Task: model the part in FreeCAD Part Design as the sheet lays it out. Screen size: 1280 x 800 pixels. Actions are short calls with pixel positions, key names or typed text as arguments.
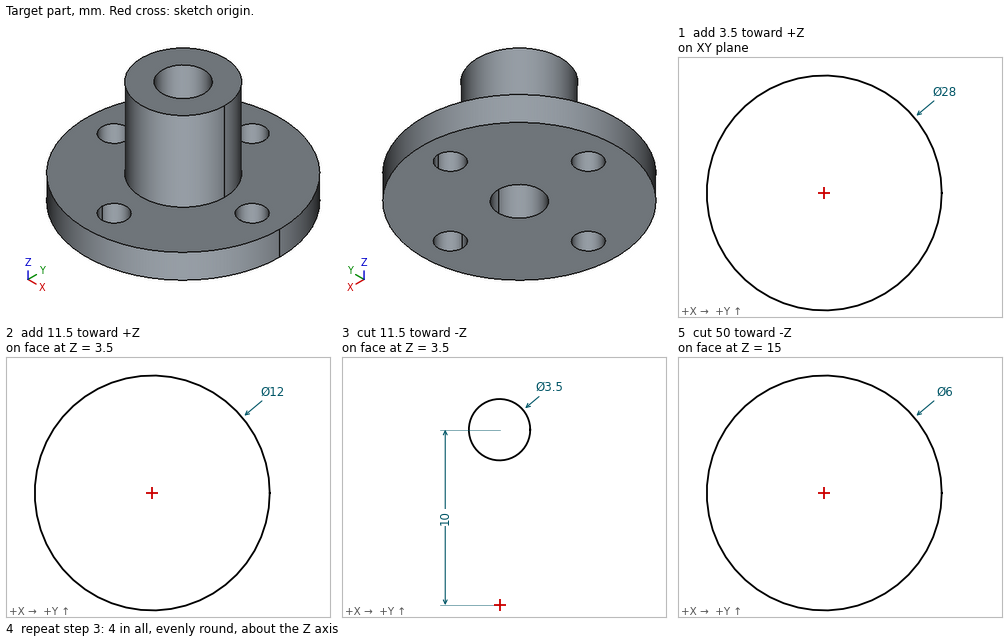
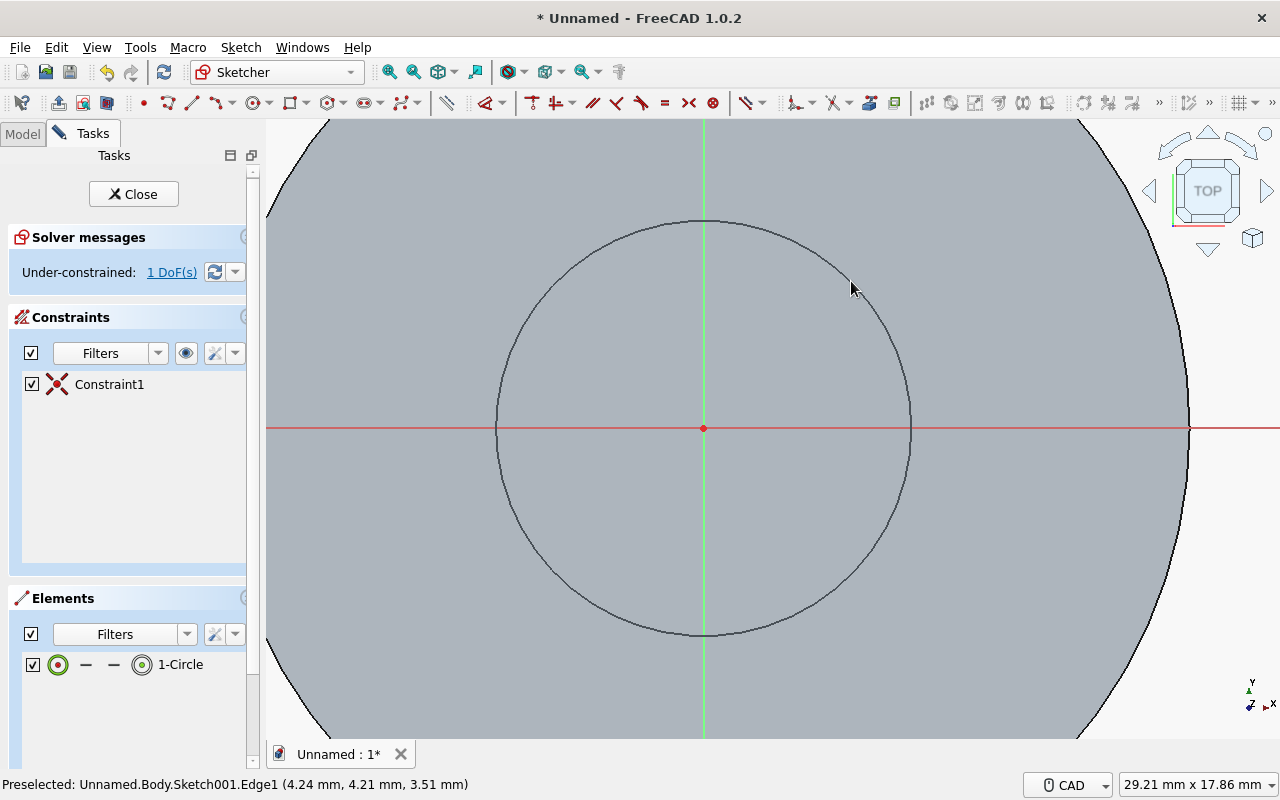
key(d)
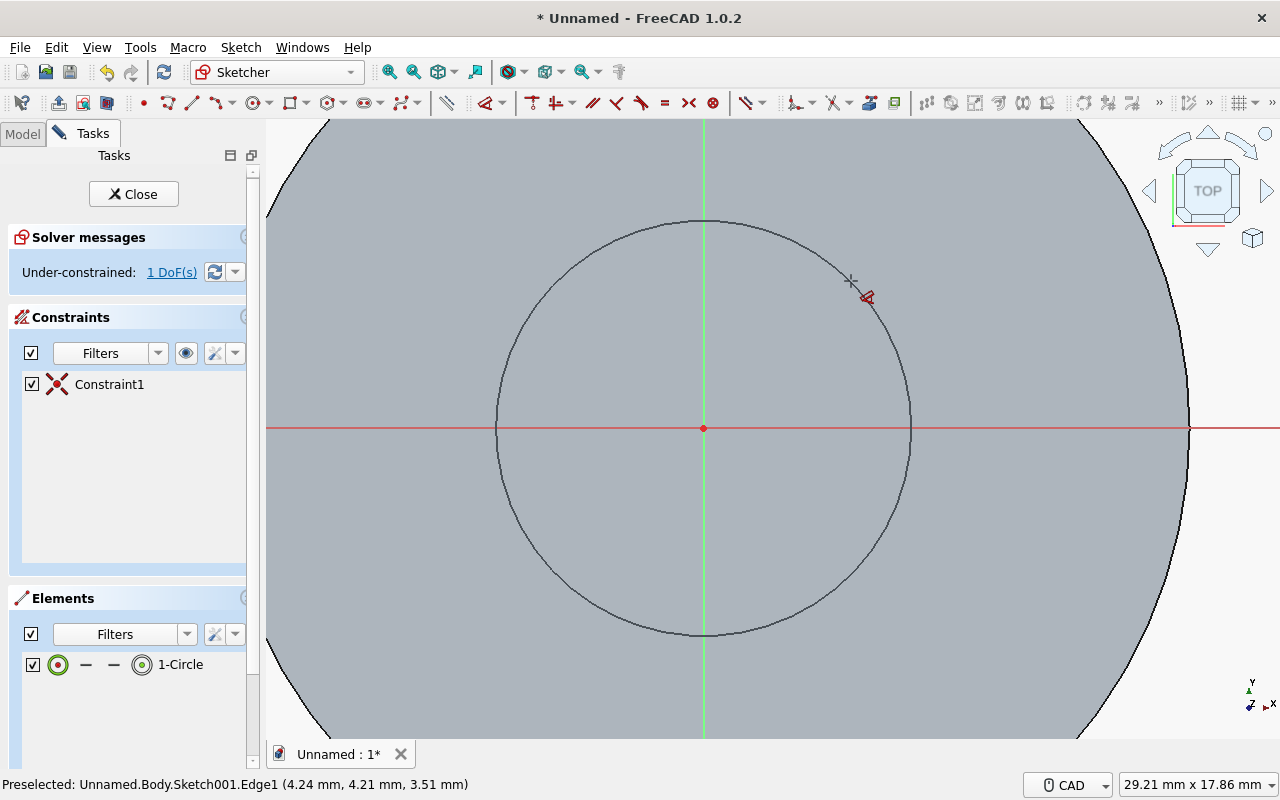
click(850, 281)
click(873, 258)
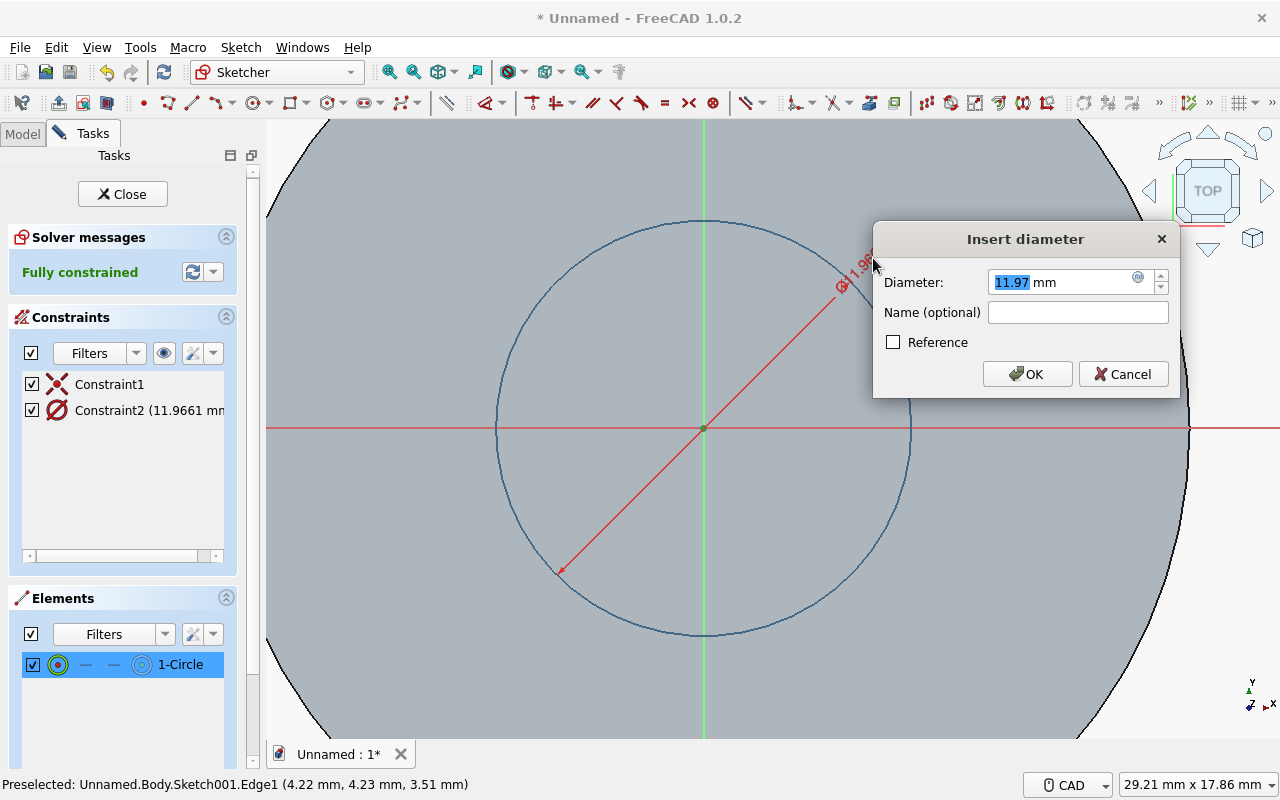
text(12)
key(Return)
key(Escape)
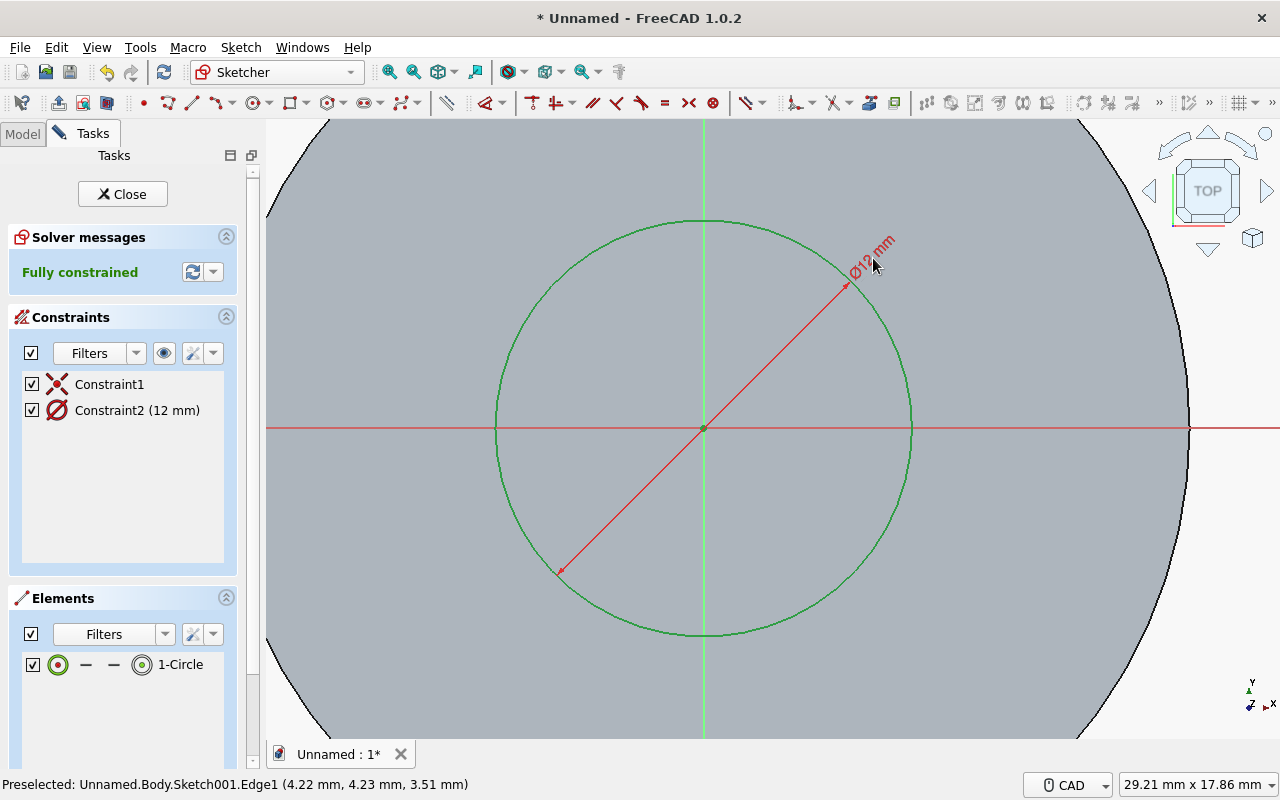
click(123, 194)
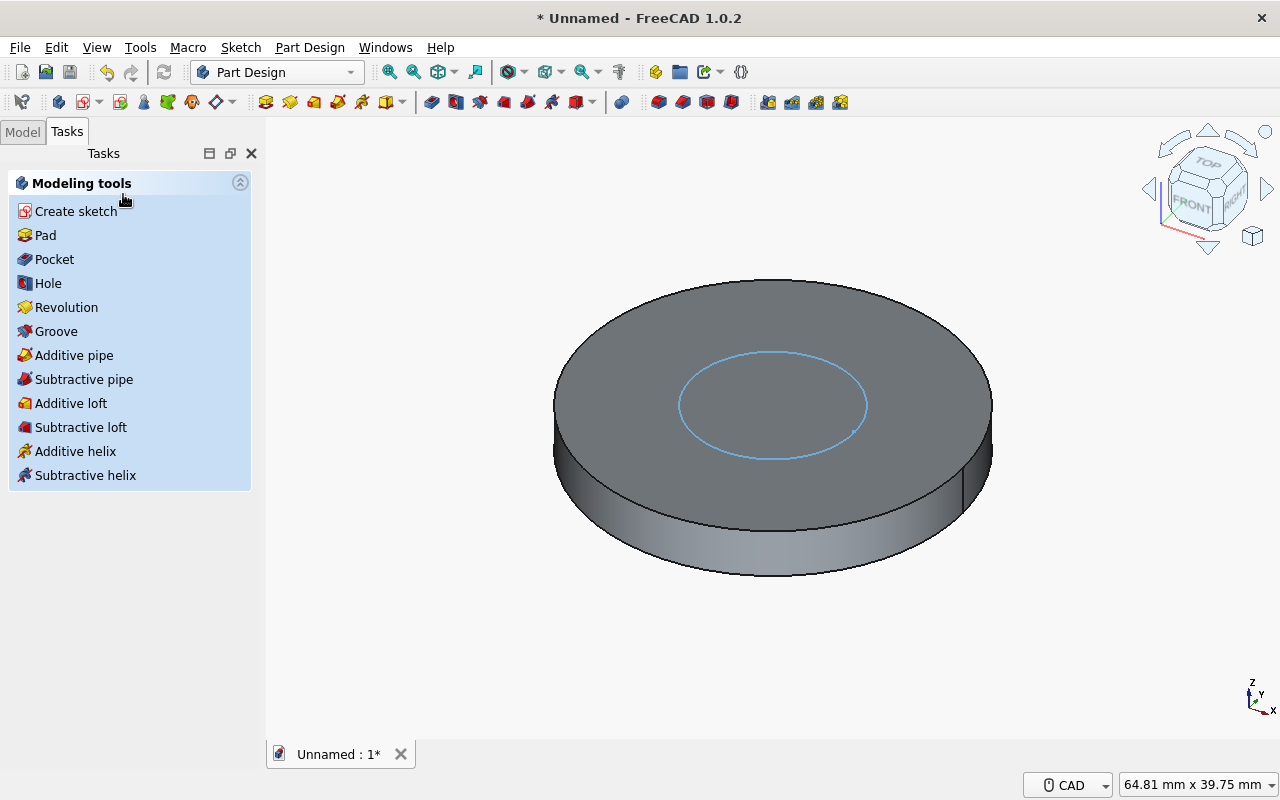
click(266, 102)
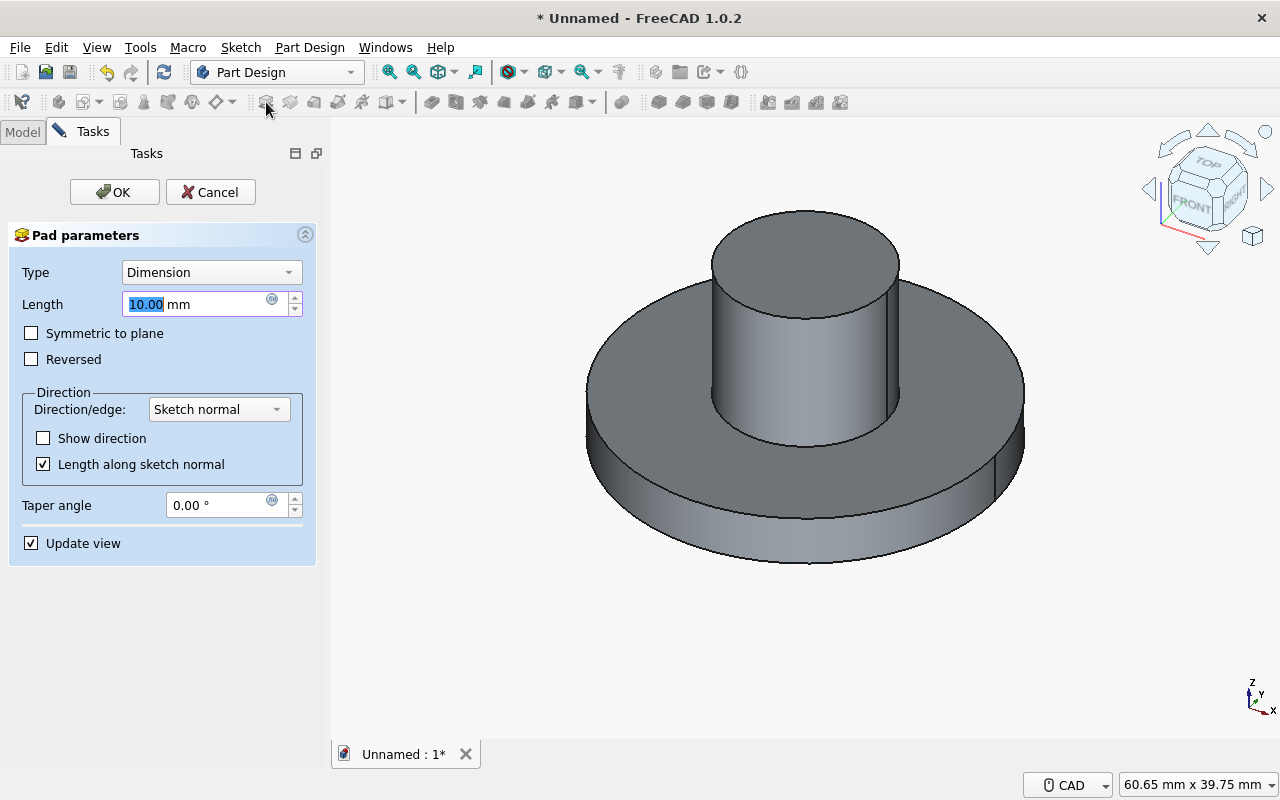
text(11.5)
key(Tab)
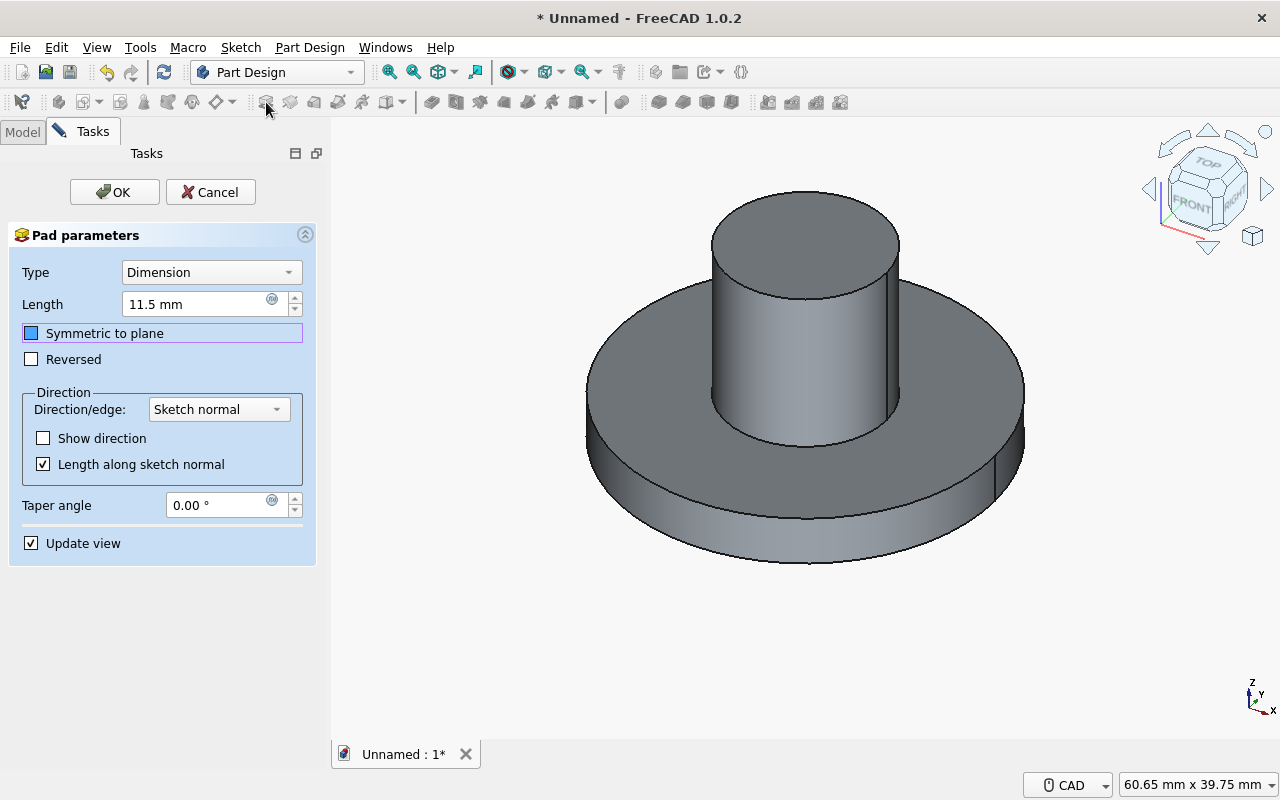
click(115, 192)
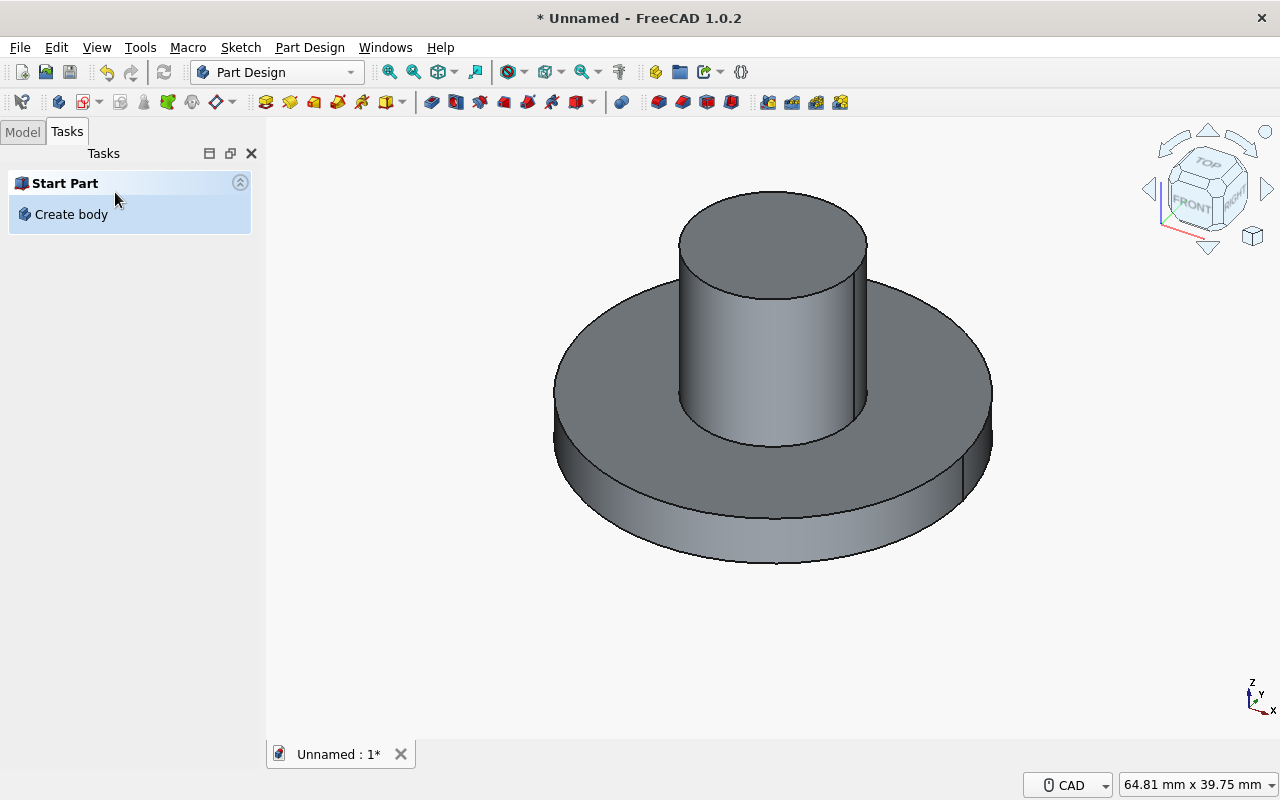
click(390, 72)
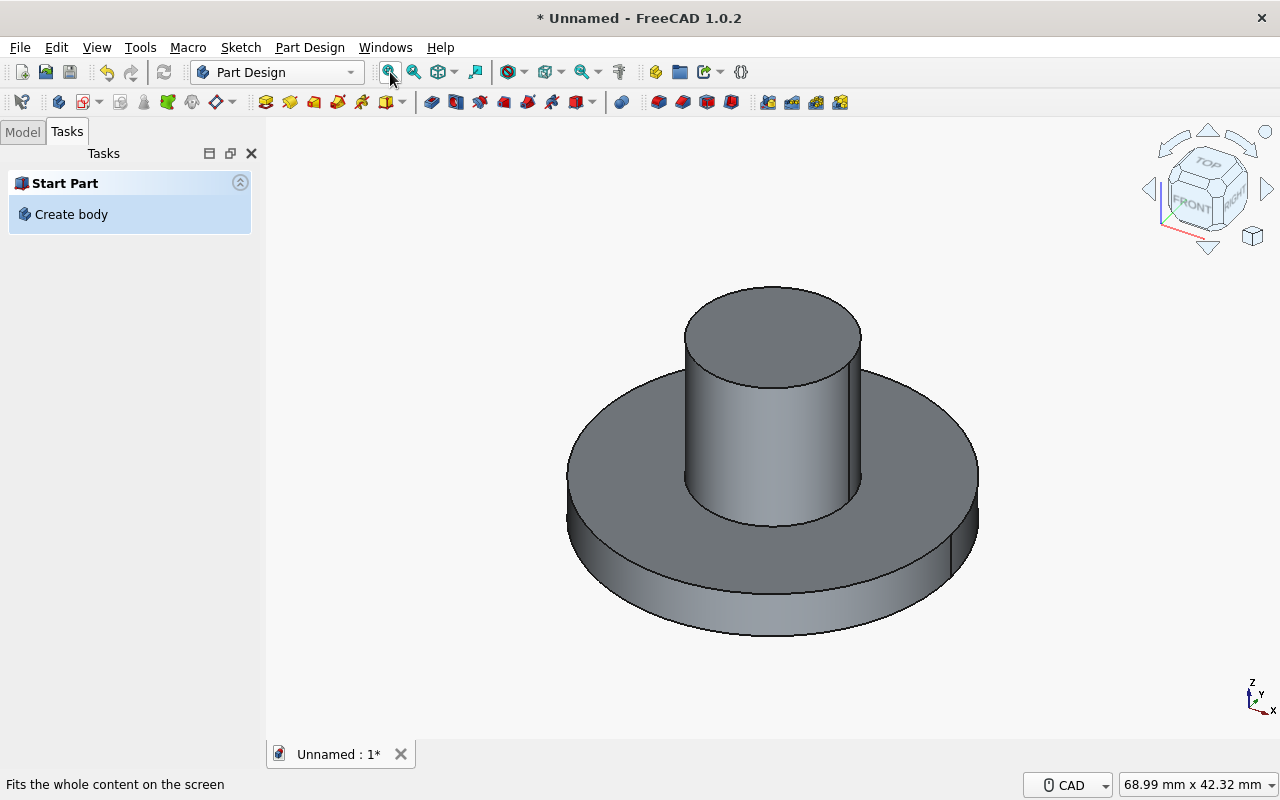
click(845, 538)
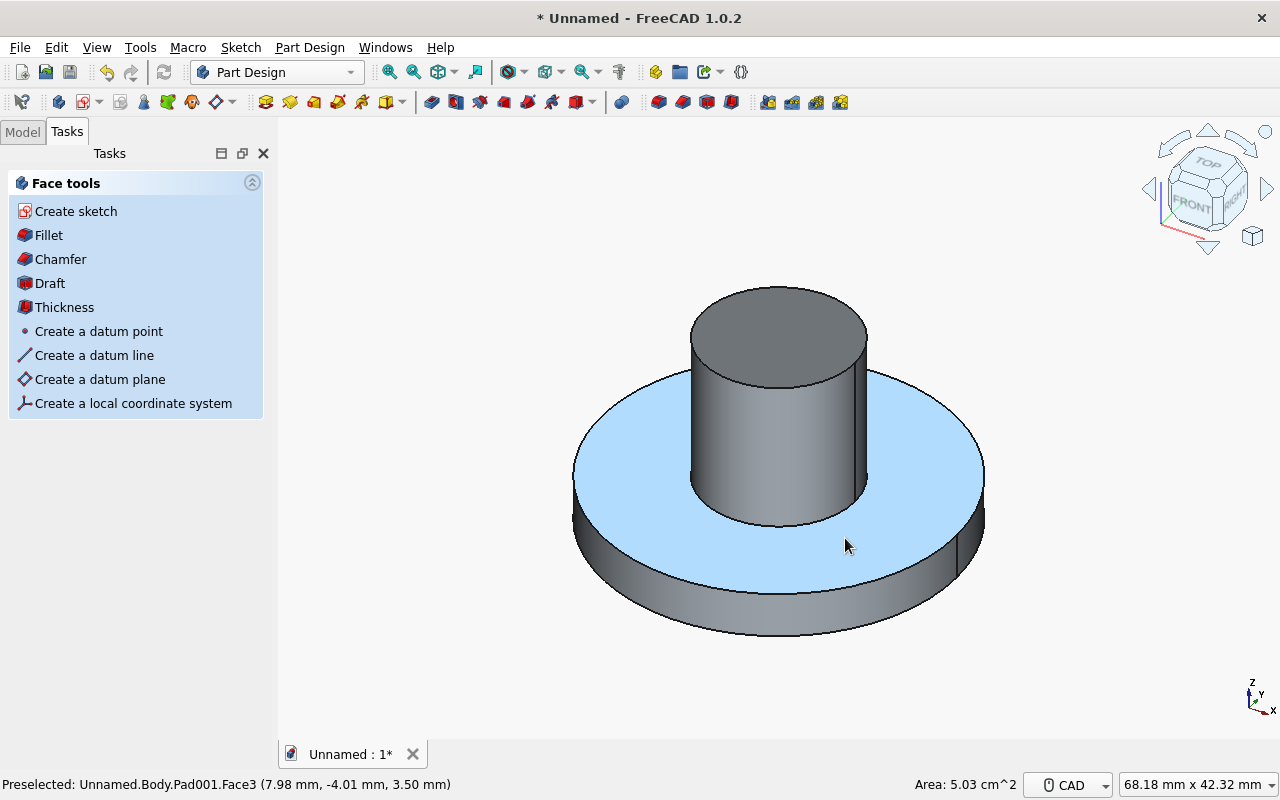
click(84, 102)